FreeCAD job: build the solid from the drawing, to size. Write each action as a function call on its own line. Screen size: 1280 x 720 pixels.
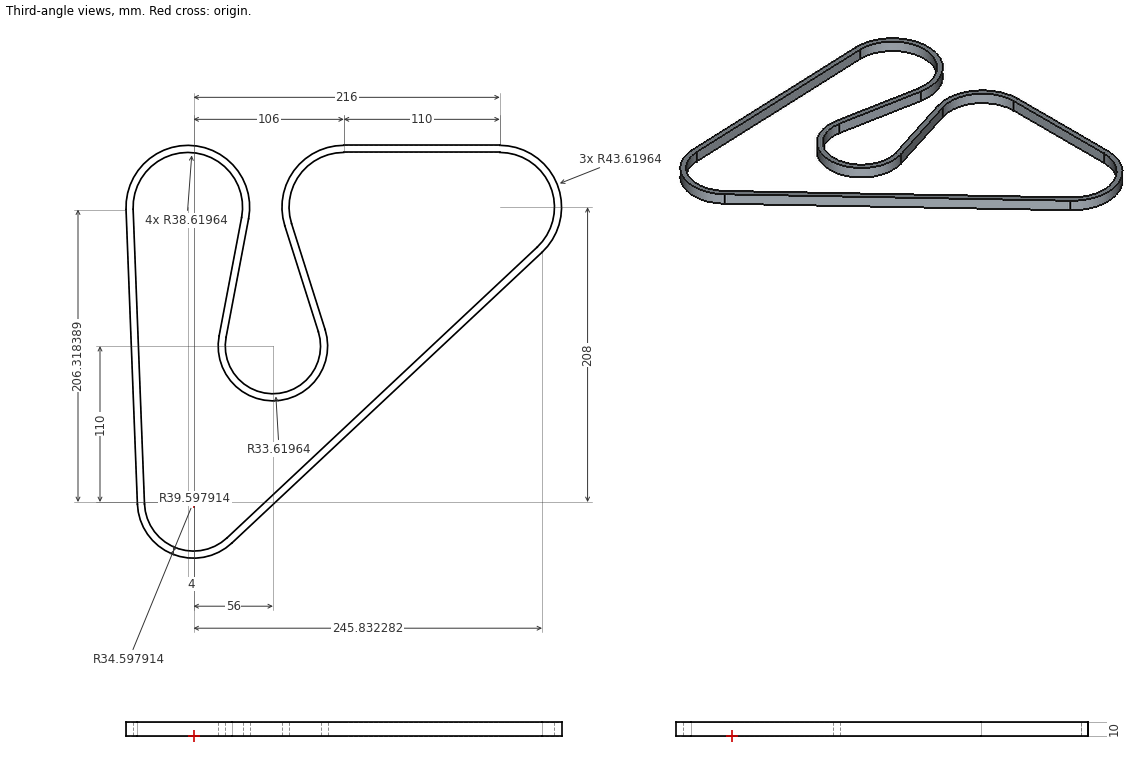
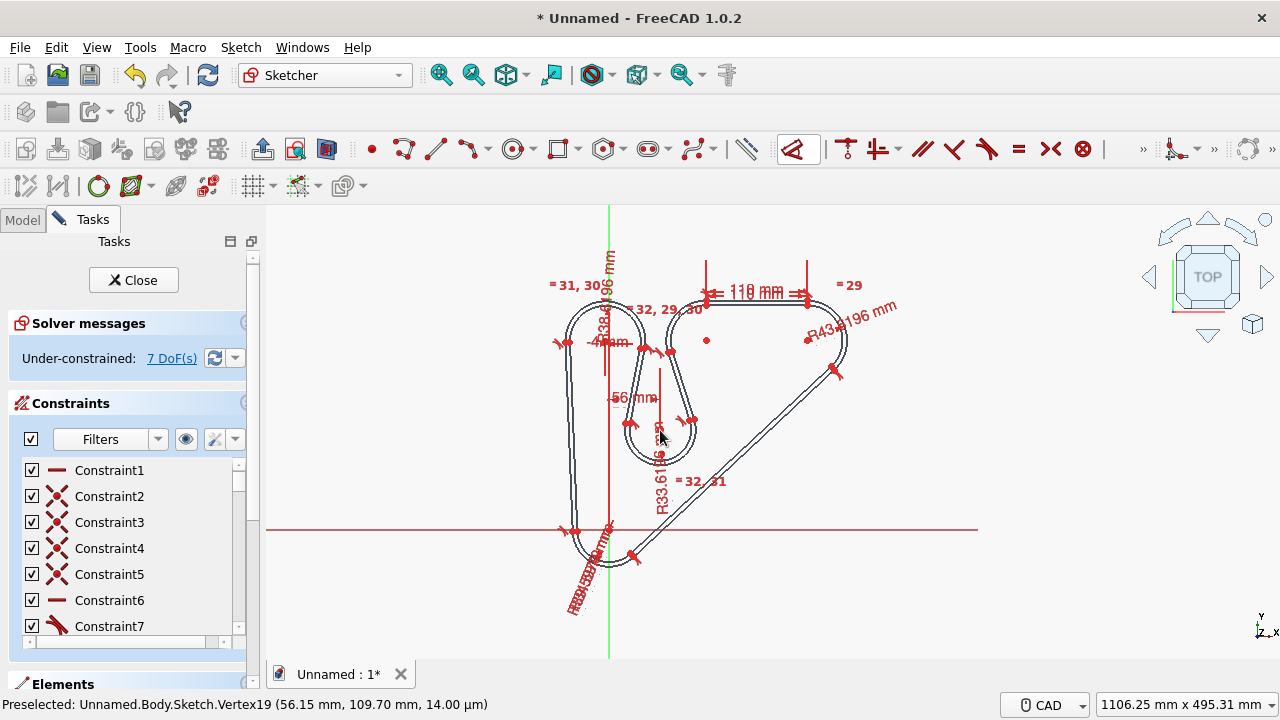
scroll(807, 301, up, 5)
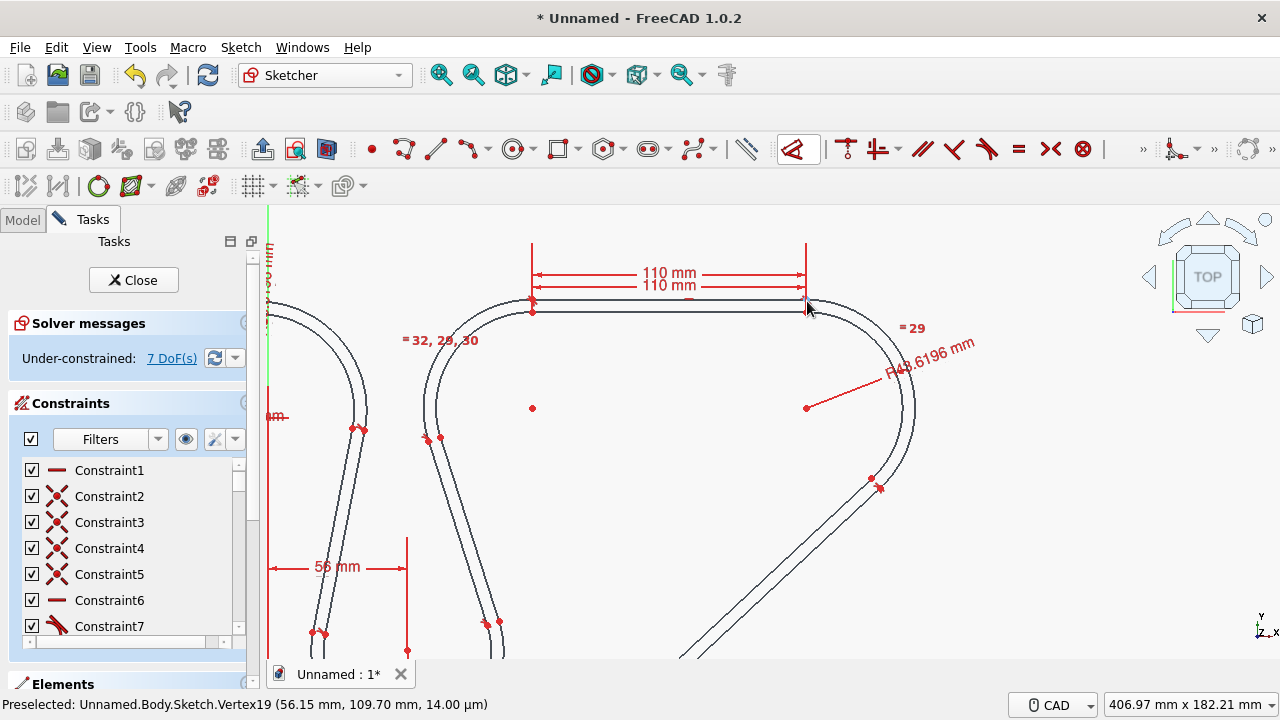
click(806, 300)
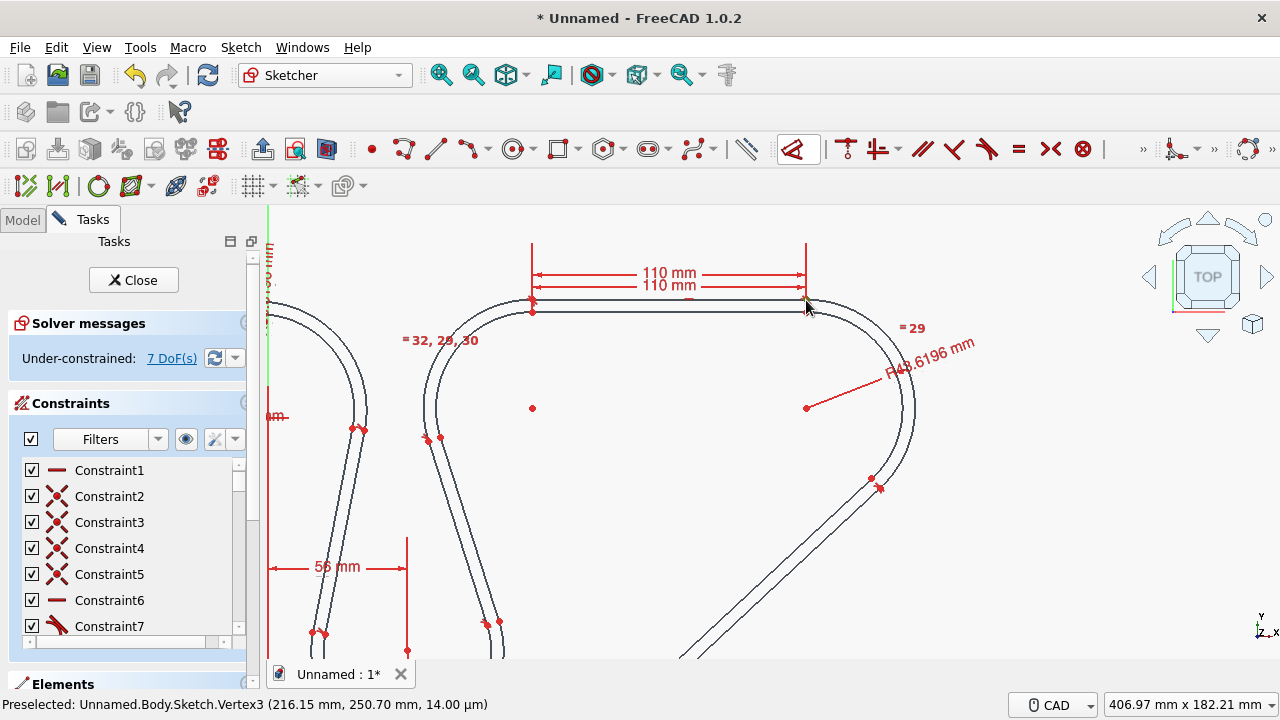
click(814, 150)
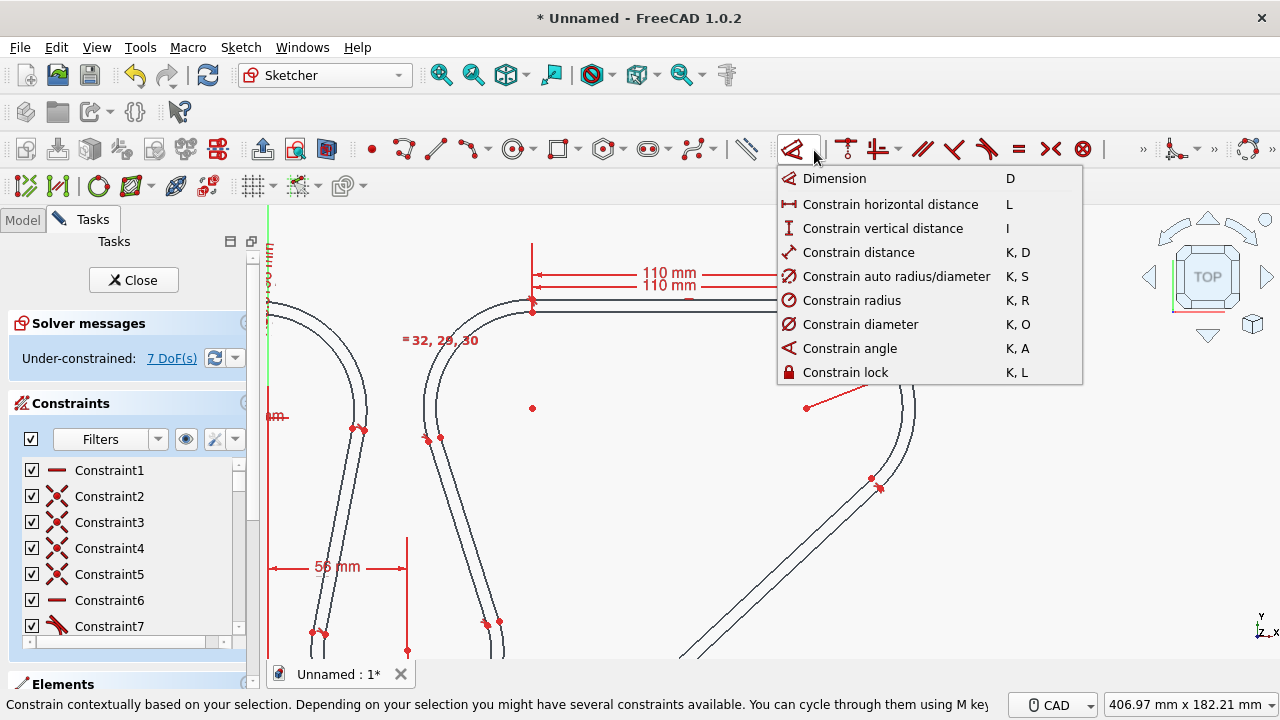
click(930, 204)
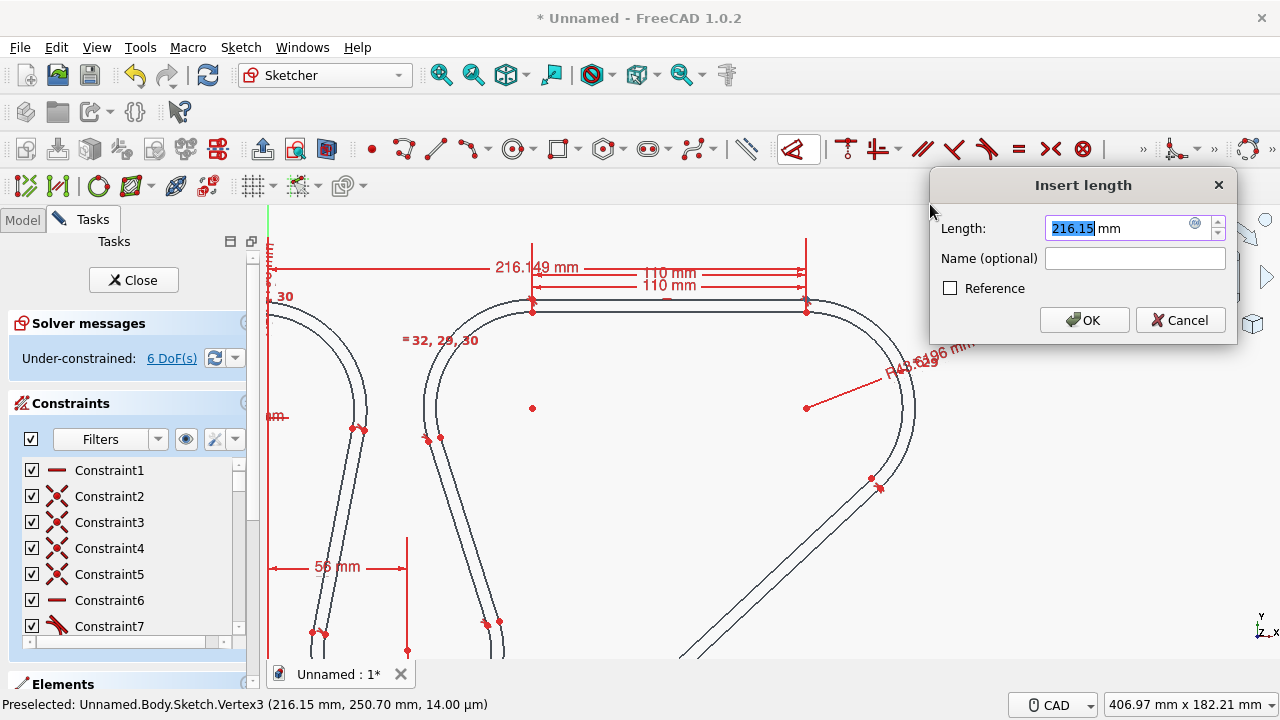
text(216)
key(Return)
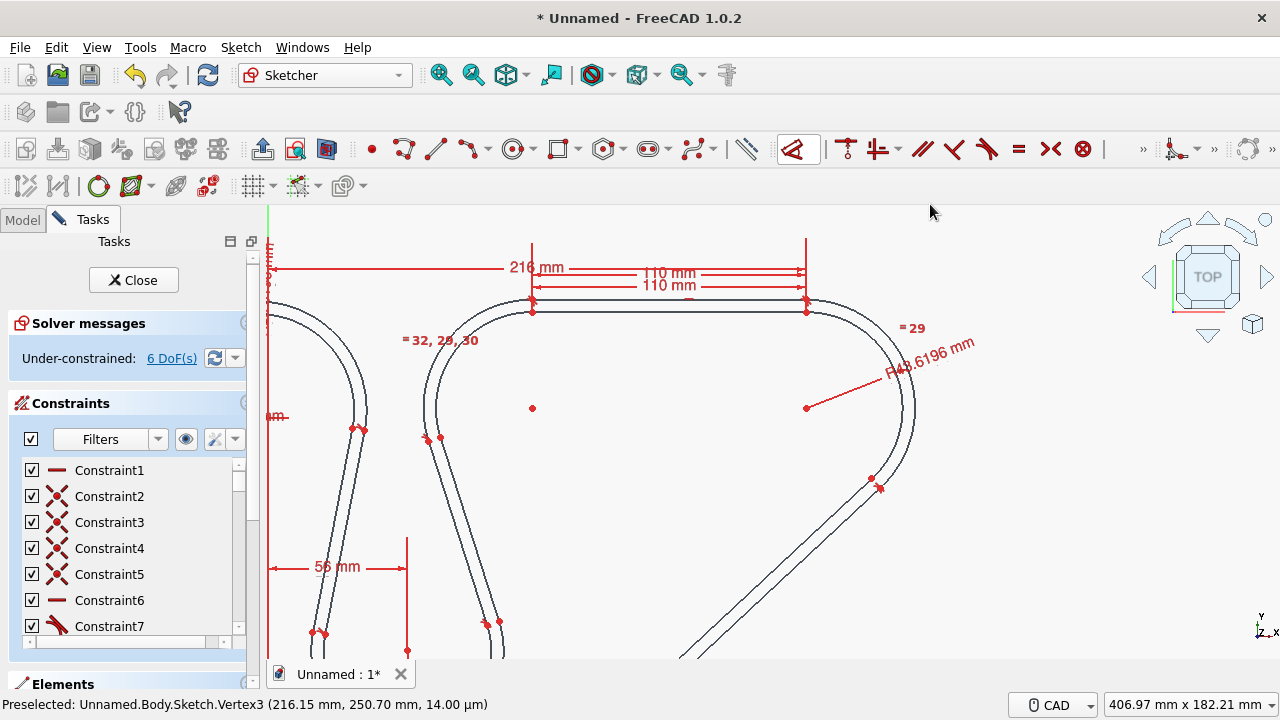
click(532, 312)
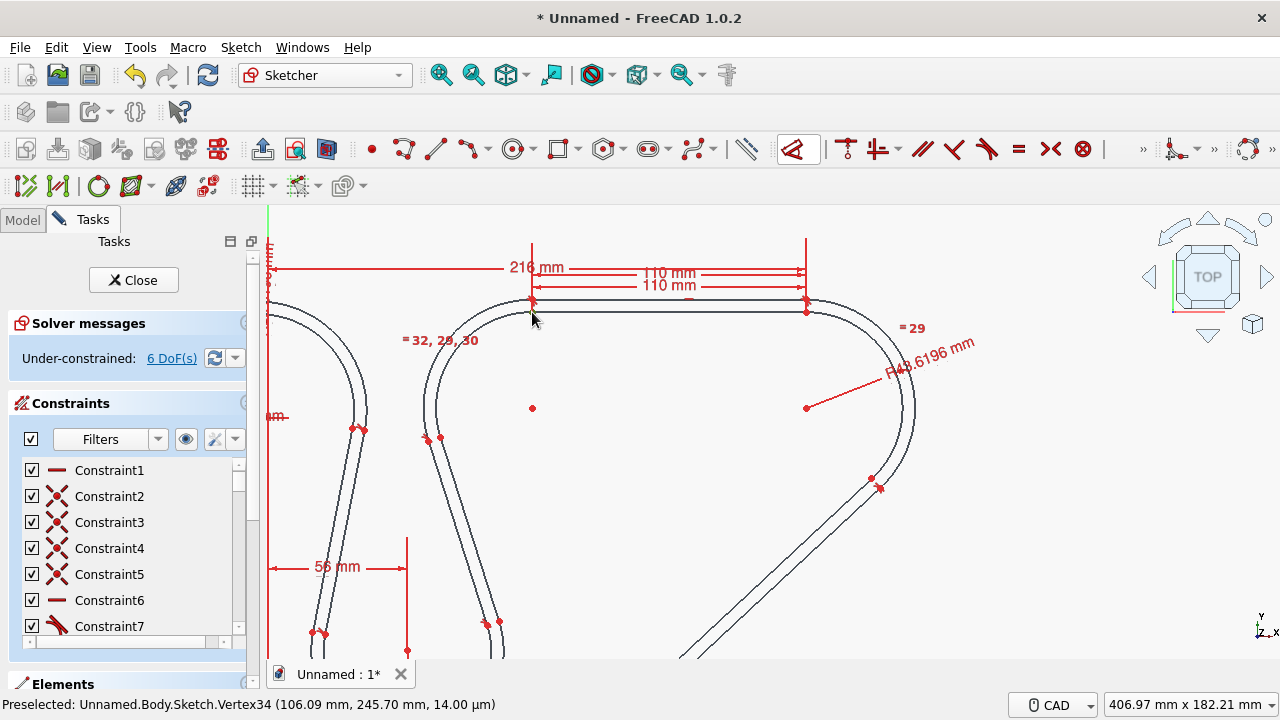
key(l)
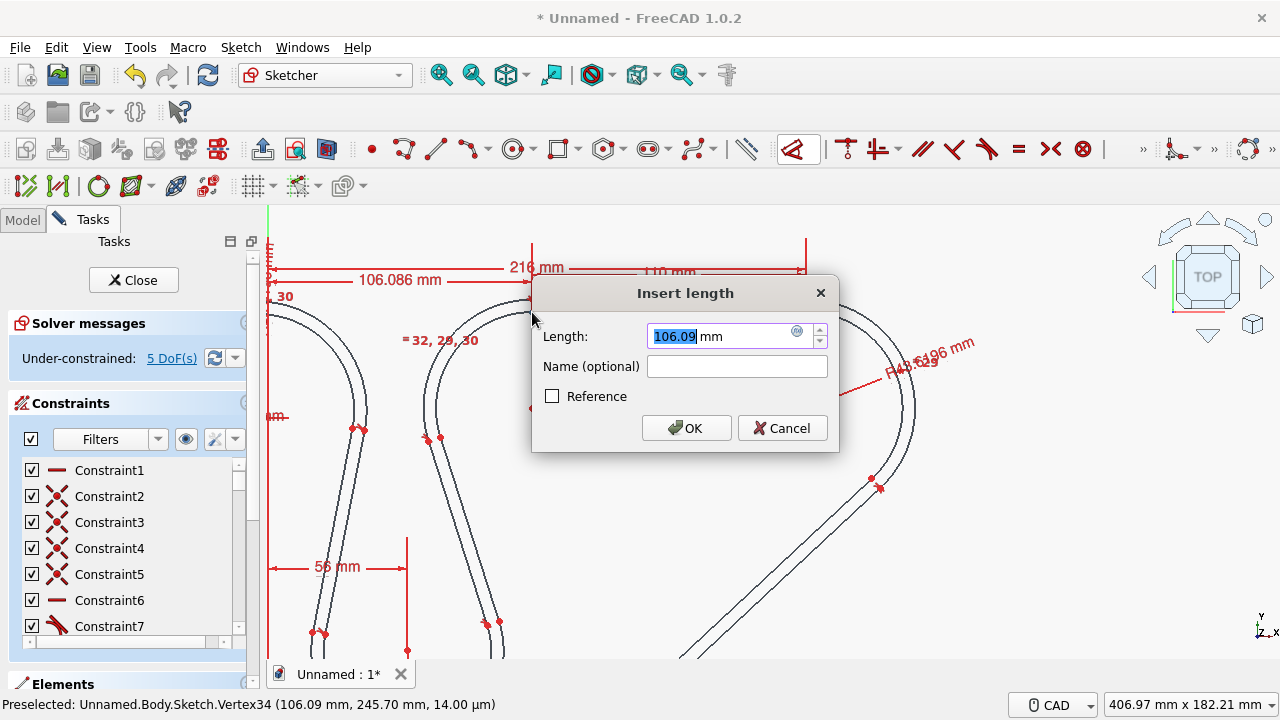
text(106)
key(Return)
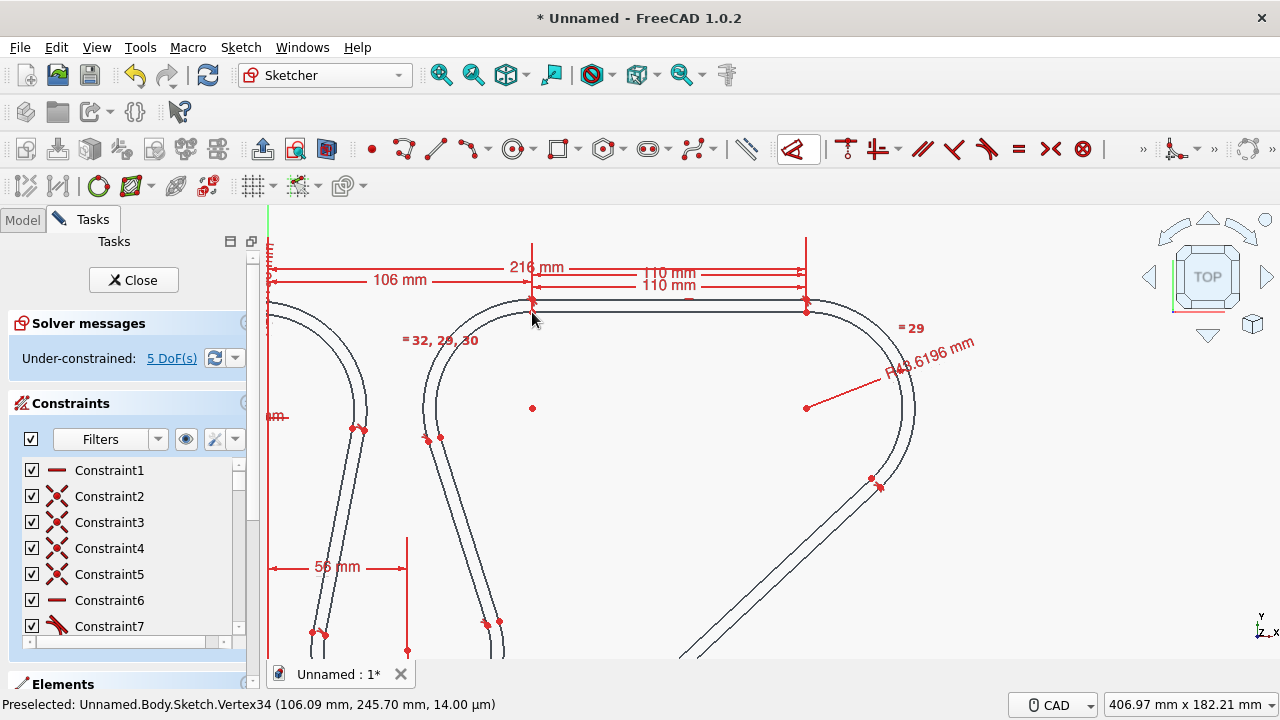
click(806, 408)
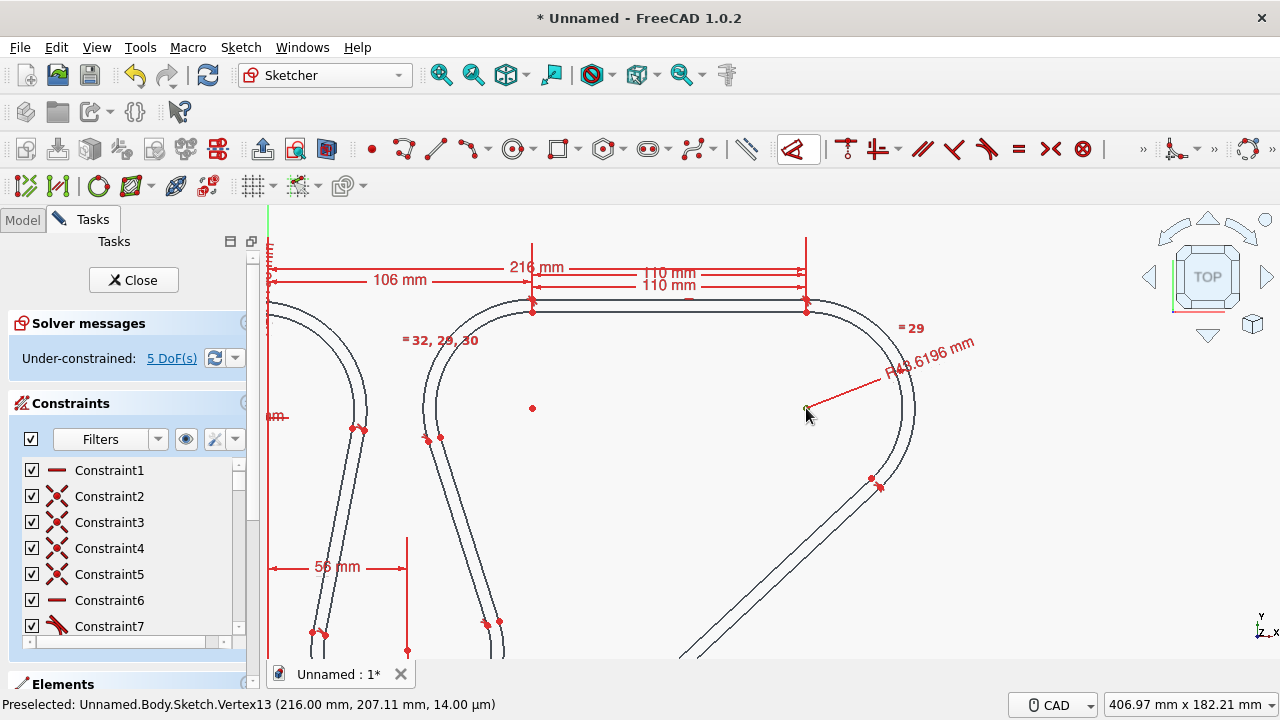
click(814, 150)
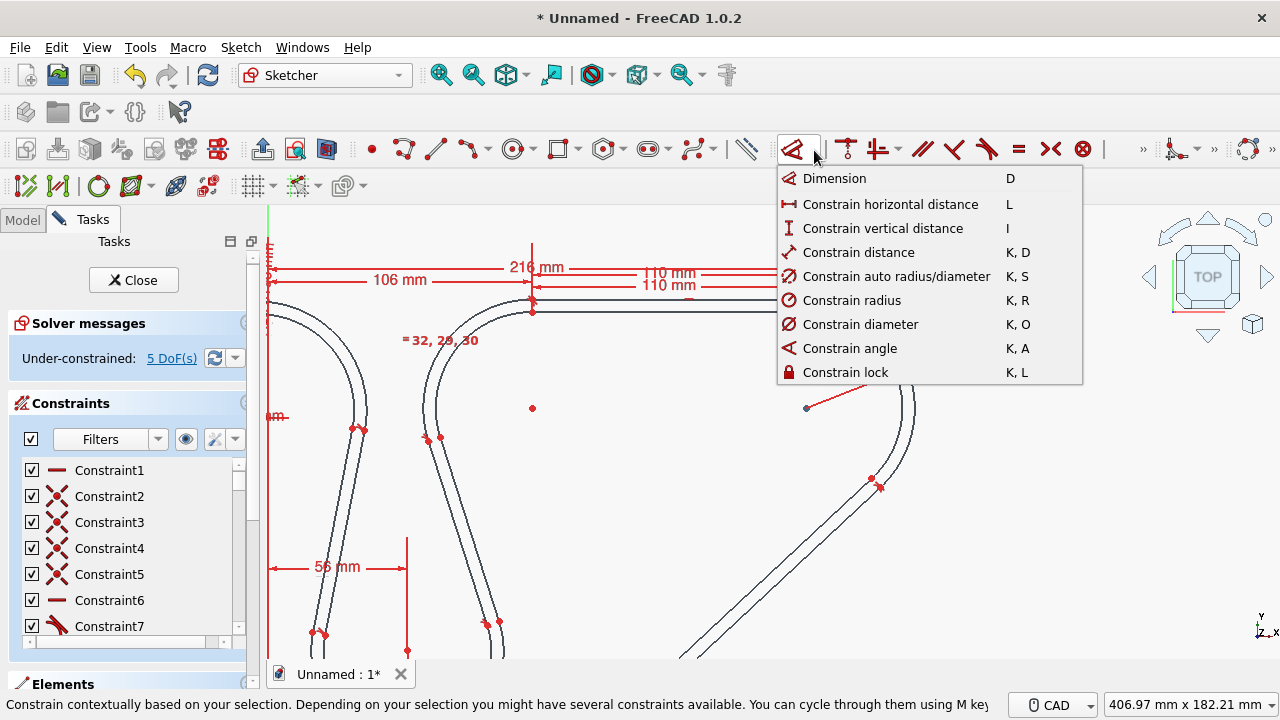
click(930, 228)